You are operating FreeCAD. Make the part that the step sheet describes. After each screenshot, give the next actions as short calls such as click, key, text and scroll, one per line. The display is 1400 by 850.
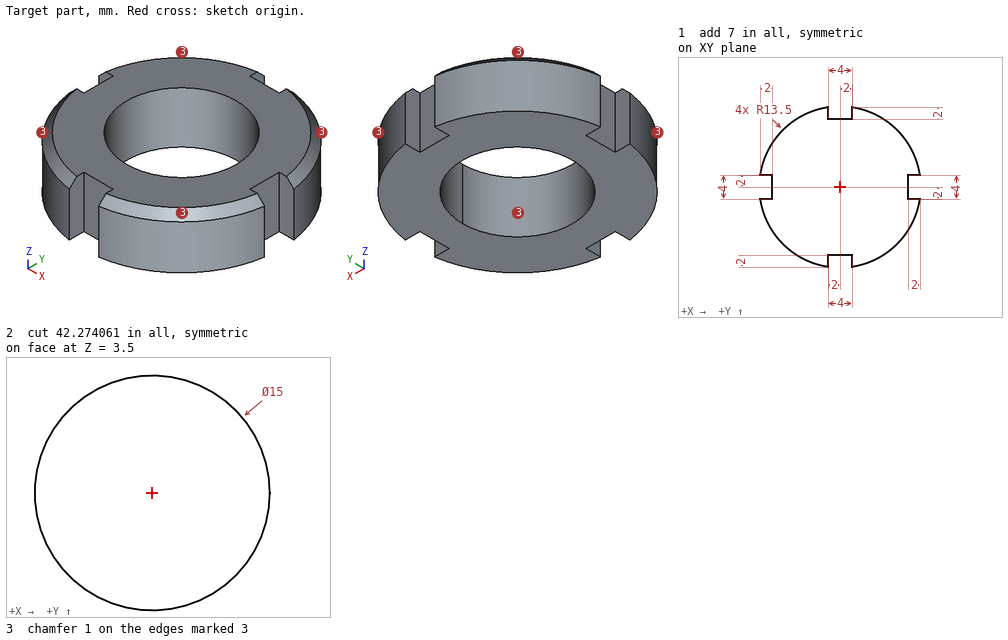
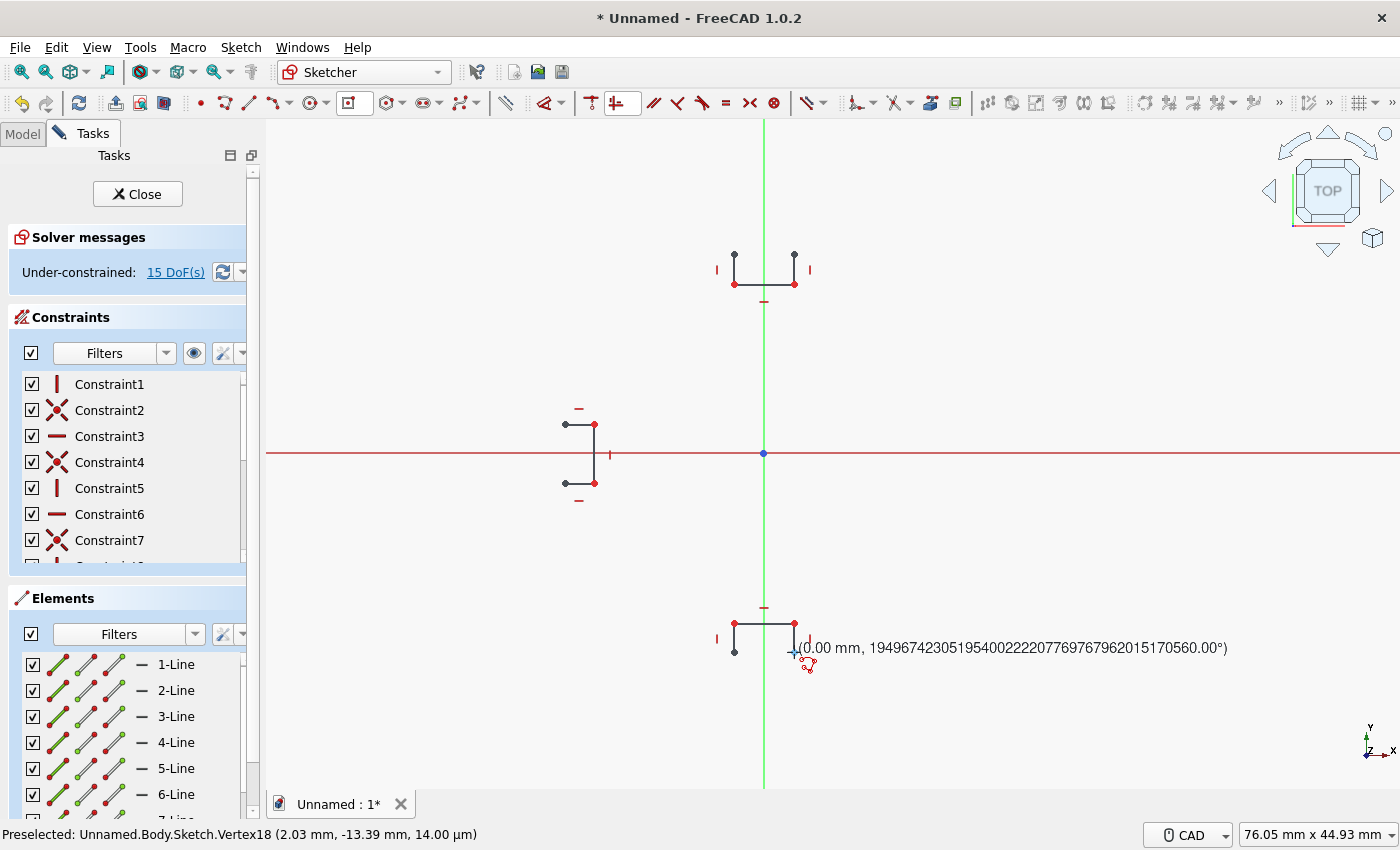
click(963, 483)
click(933, 483)
click(933, 424)
click(963, 424)
right_click(963, 424)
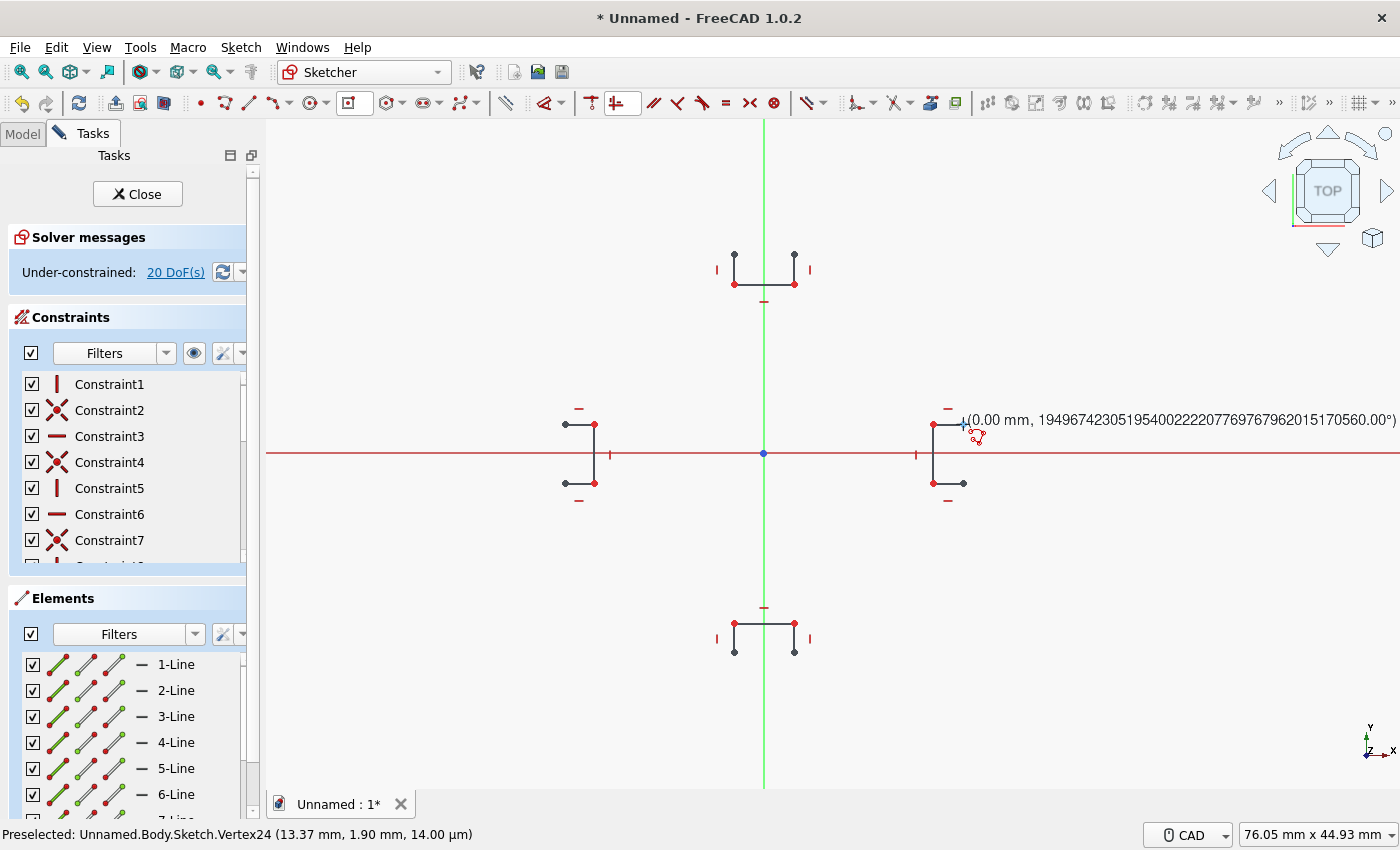
key(g)
key(3)
key(a)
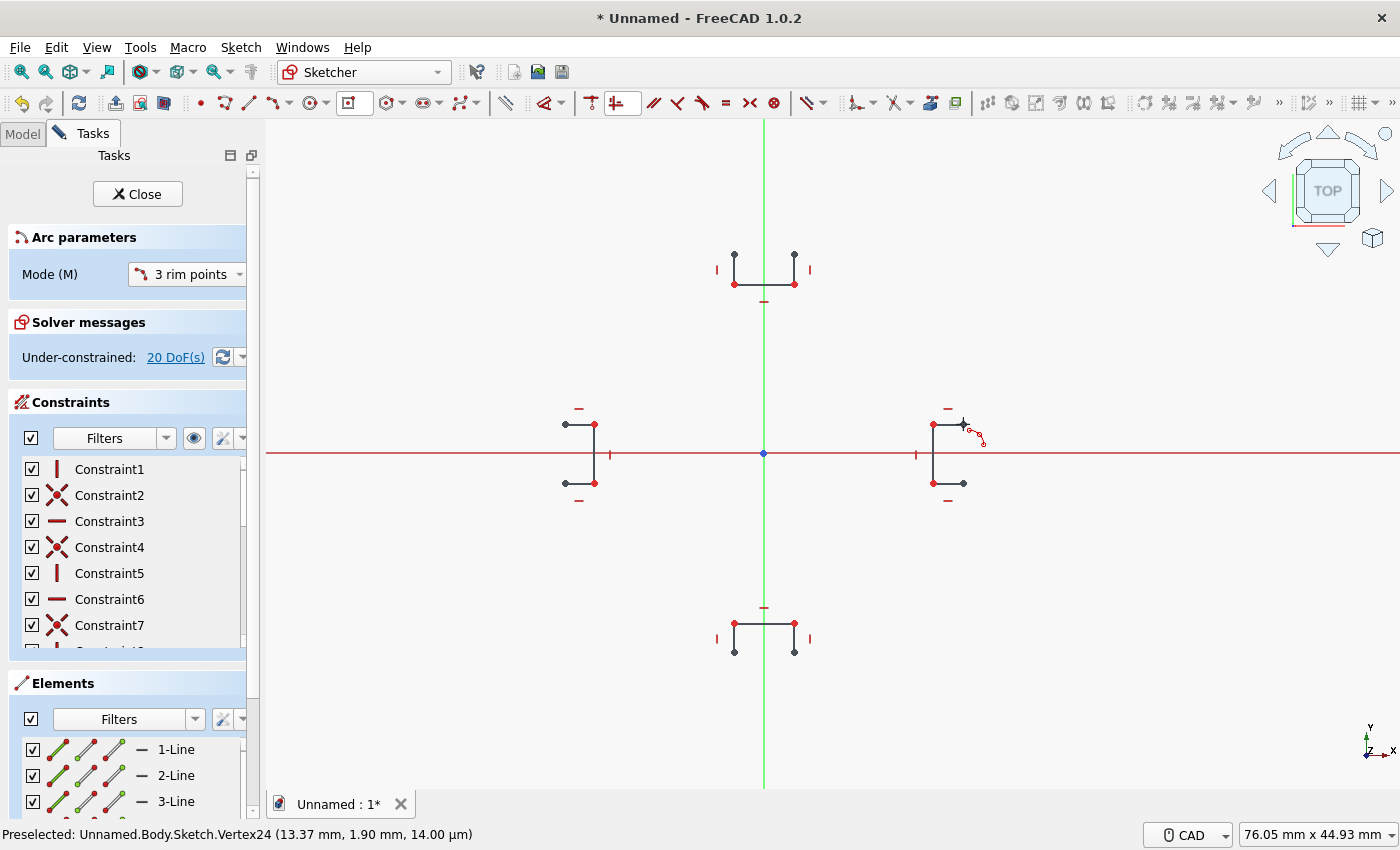
click(734, 255)
click(565, 425)
click(621, 311)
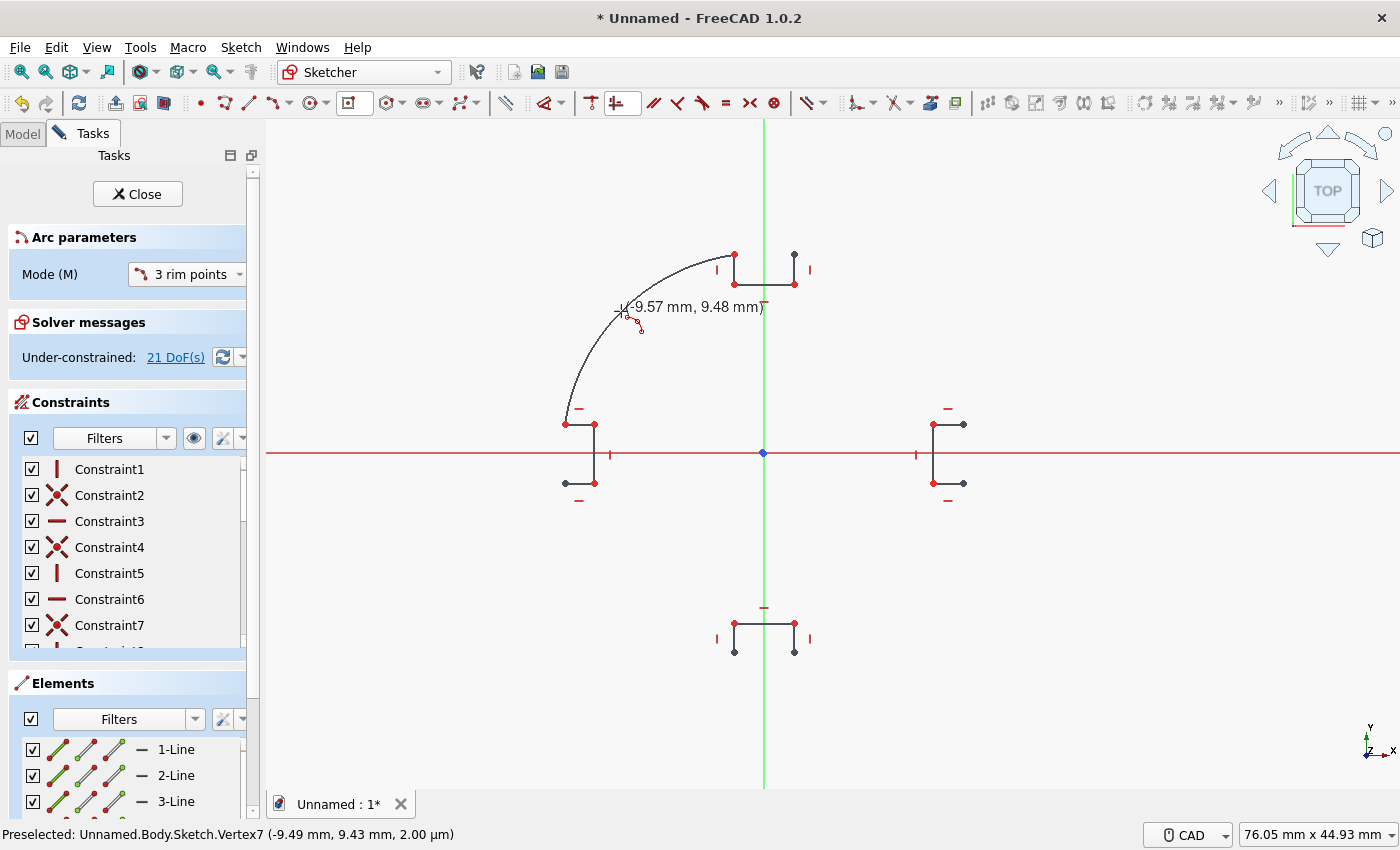
click(565, 484)
click(734, 653)
click(621, 596)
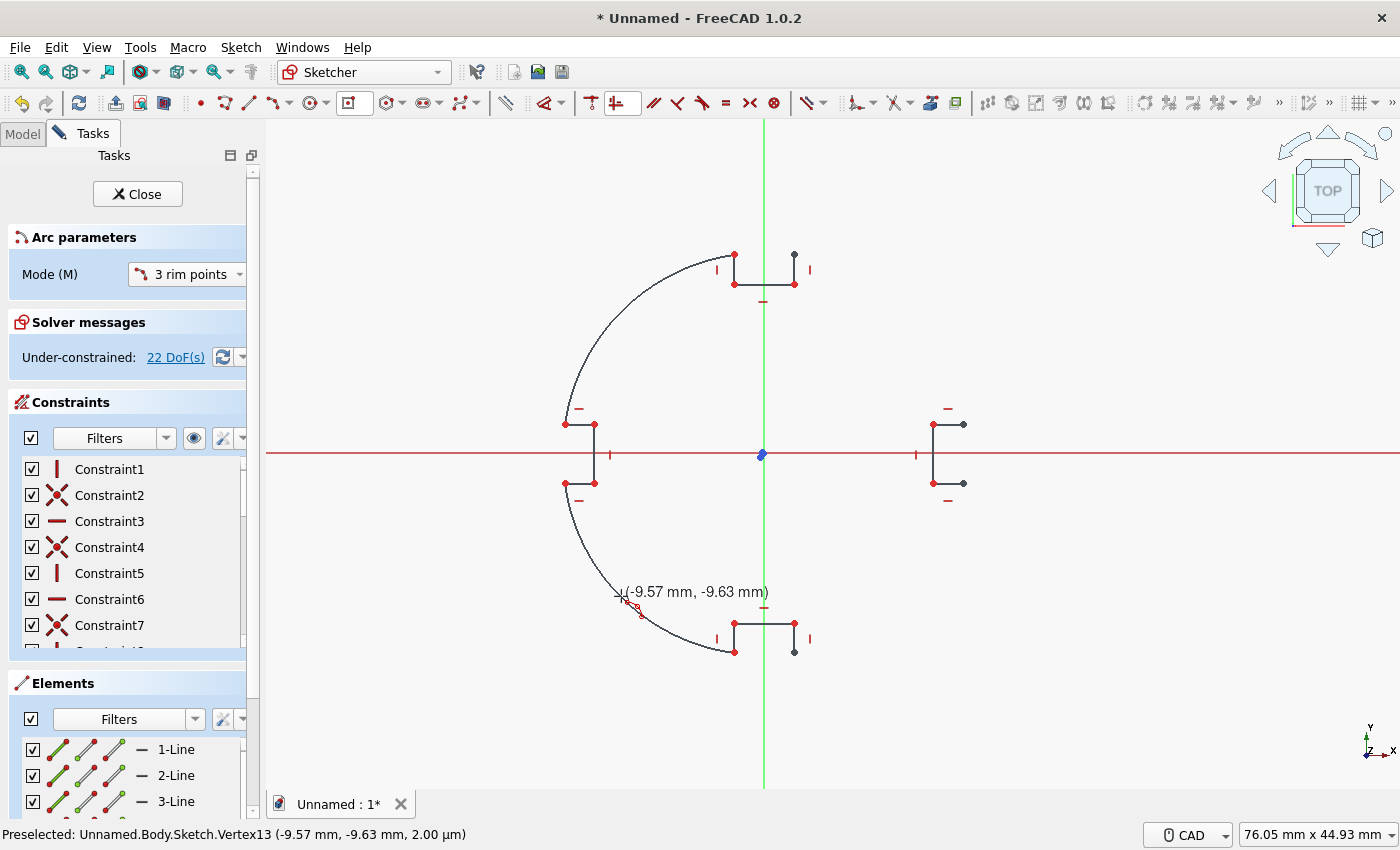
click(794, 653)
click(963, 484)
click(906, 596)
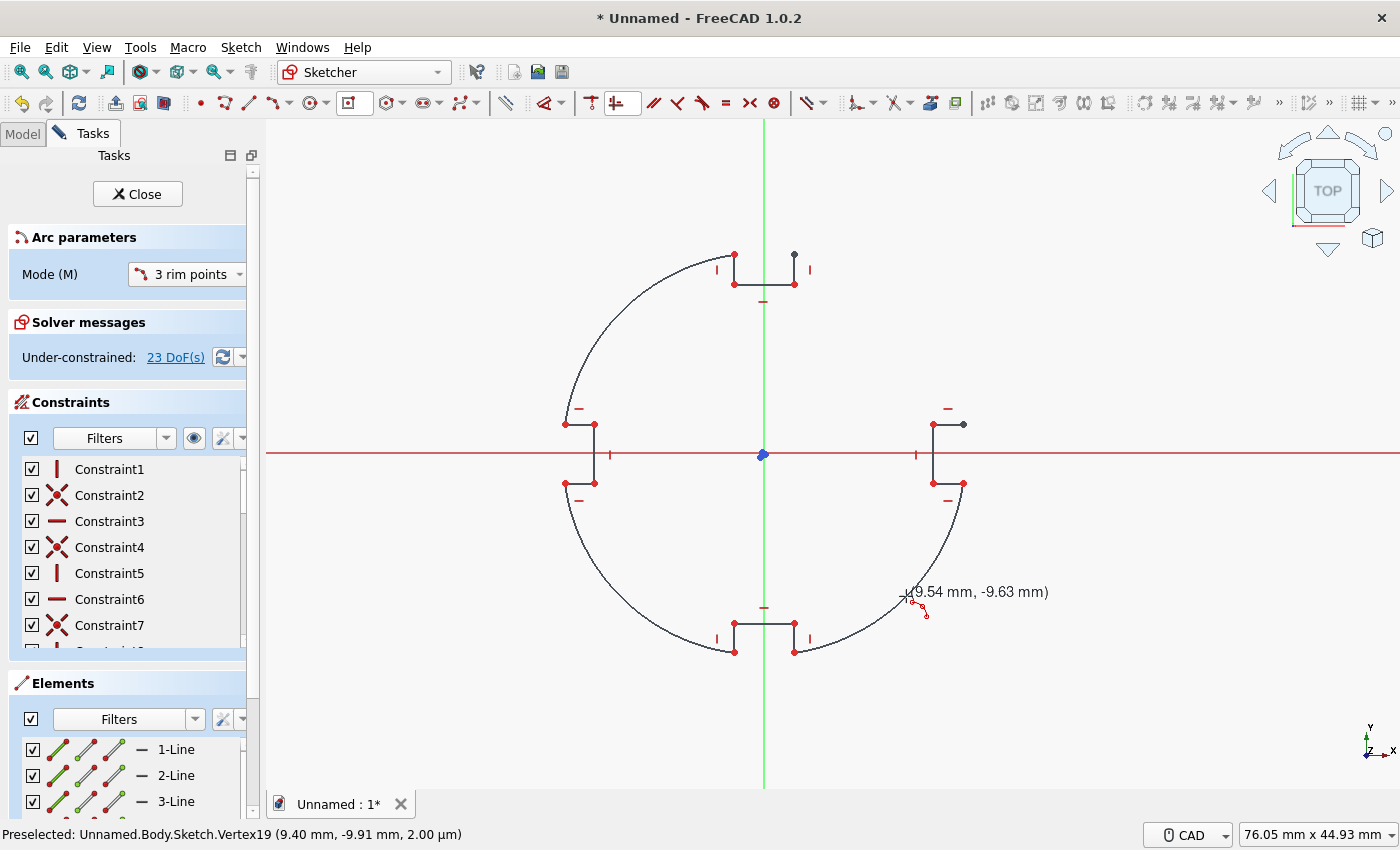
click(963, 425)
click(794, 255)
click(906, 311)
key(Escape)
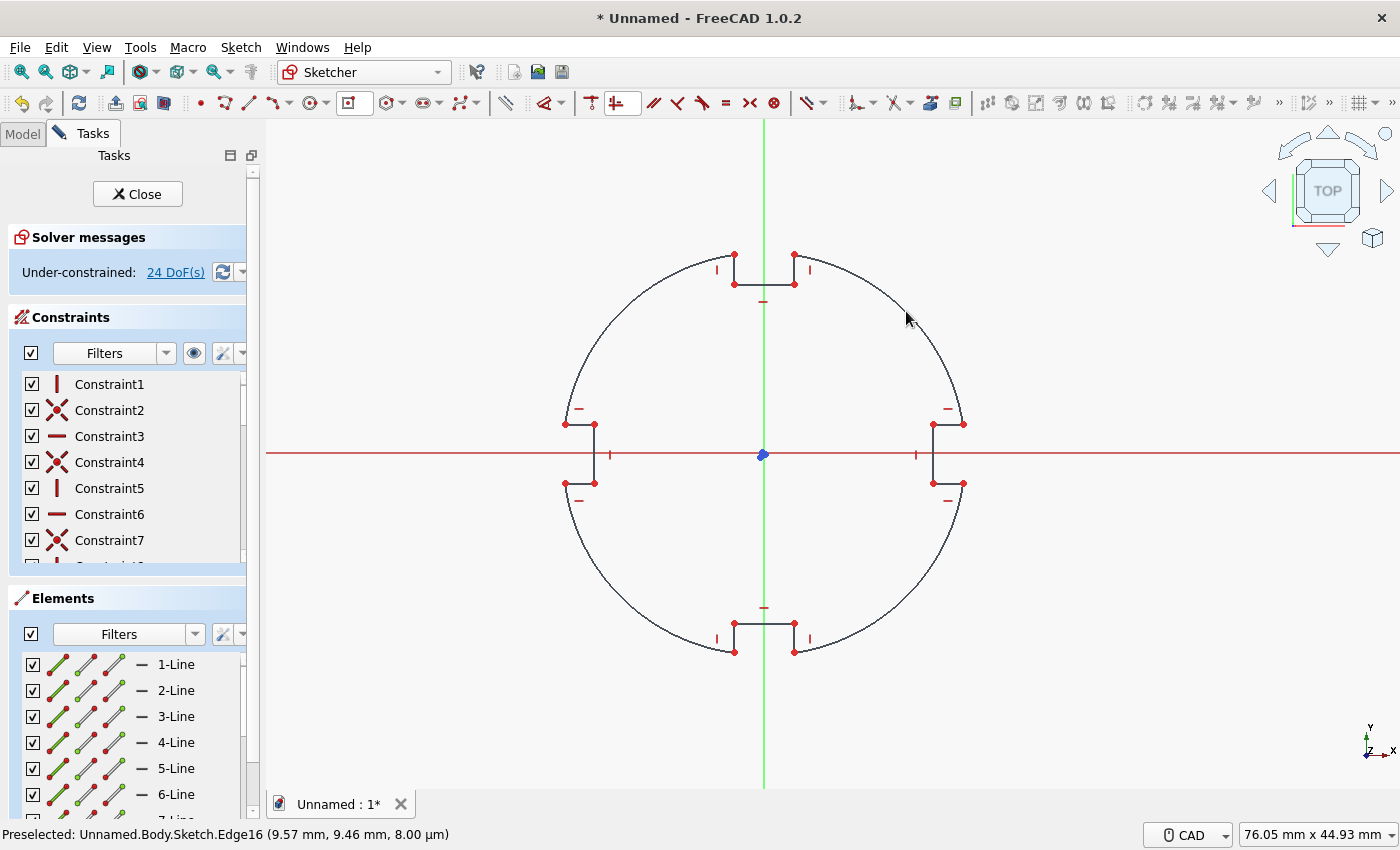
click(662, 280)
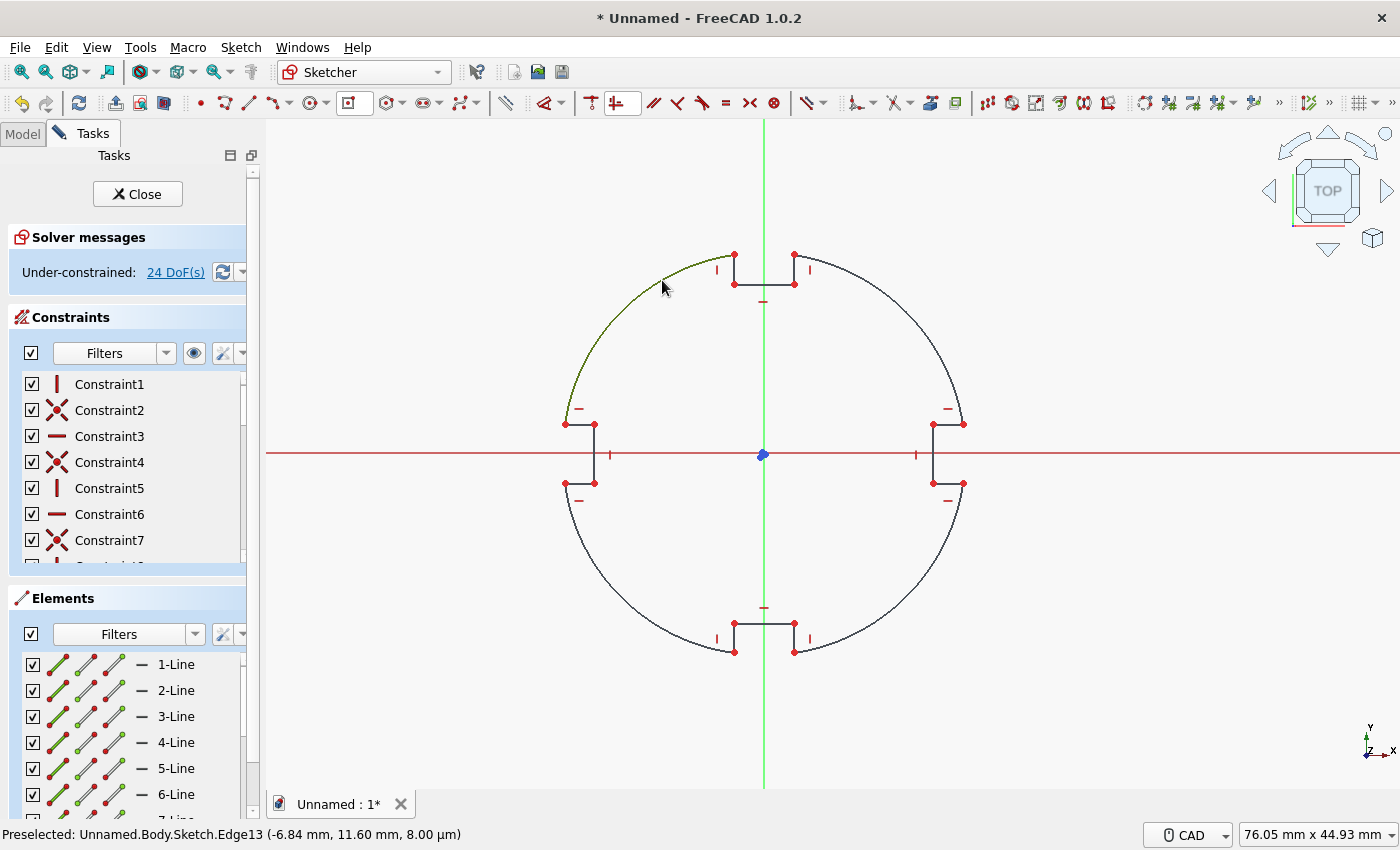
click(590, 556)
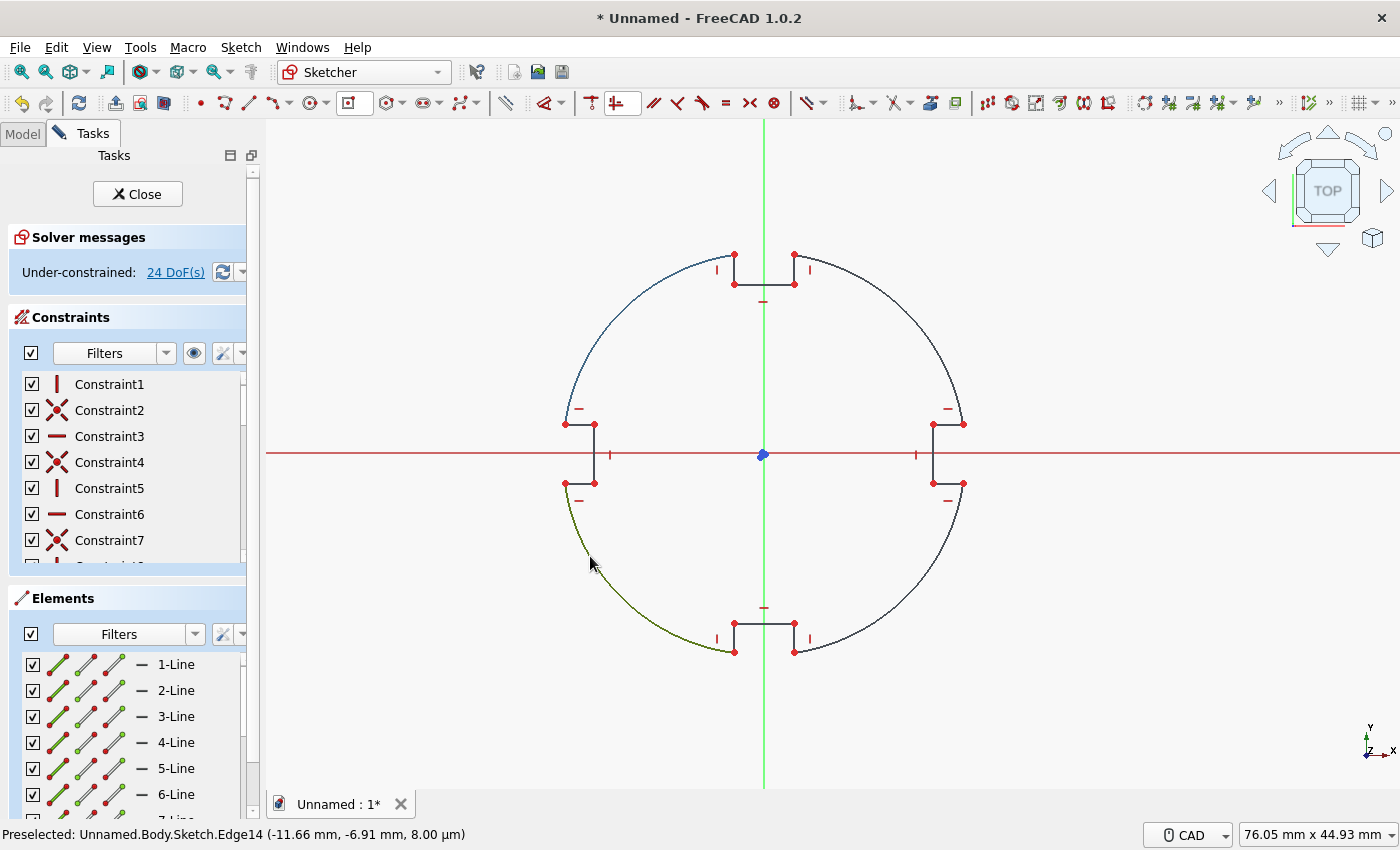
click(592, 104)